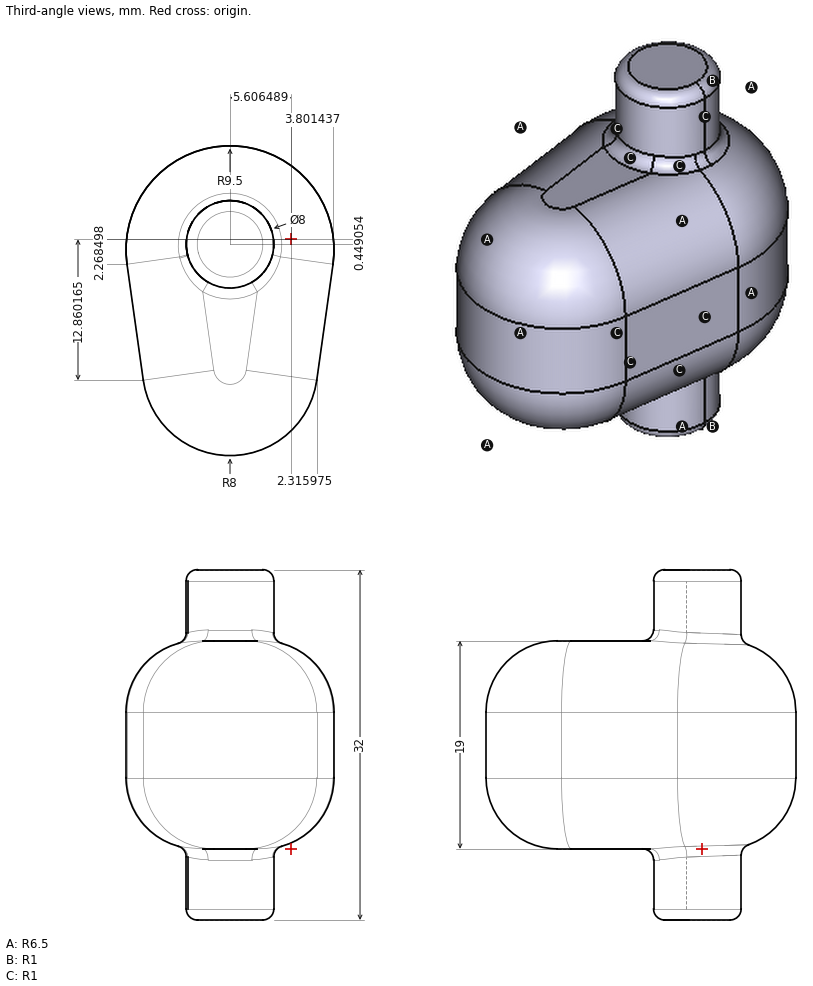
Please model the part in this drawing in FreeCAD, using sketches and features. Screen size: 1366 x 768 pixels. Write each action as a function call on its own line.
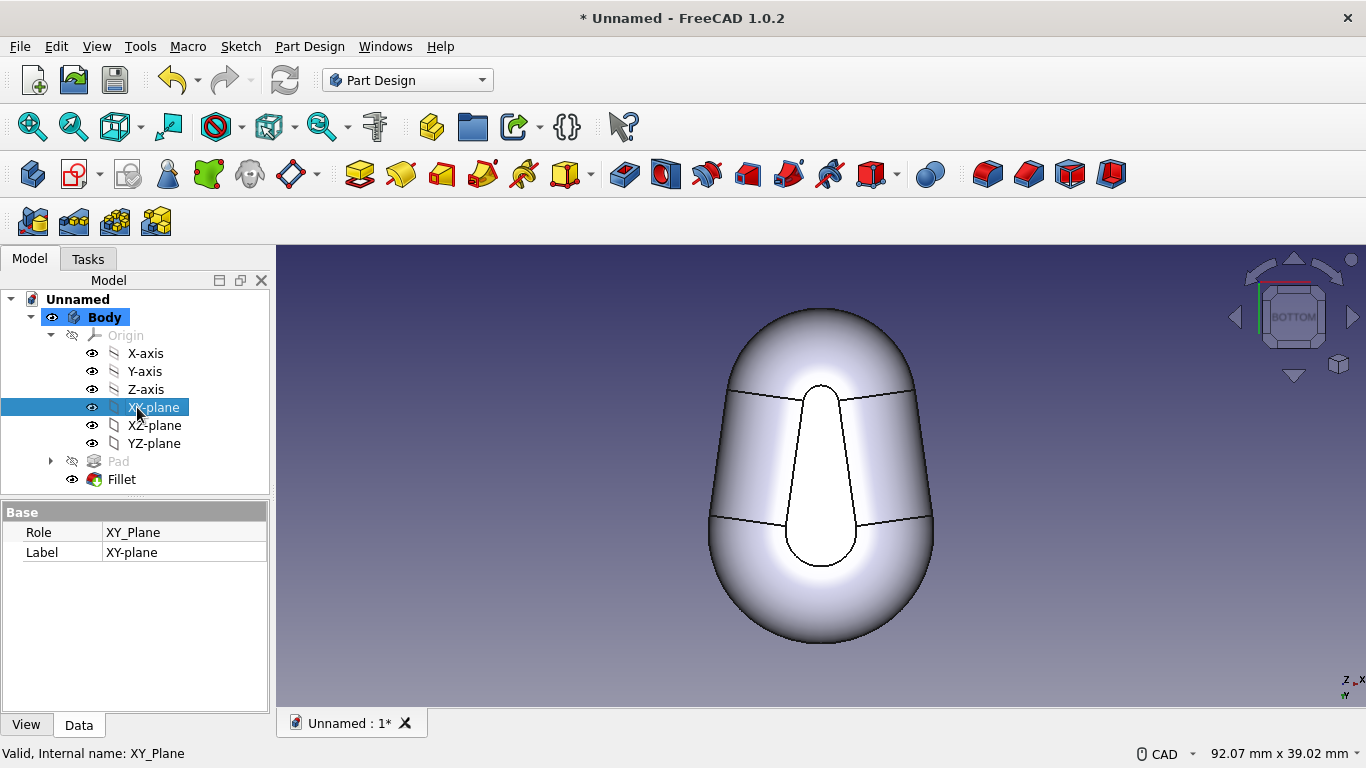
click(290, 174)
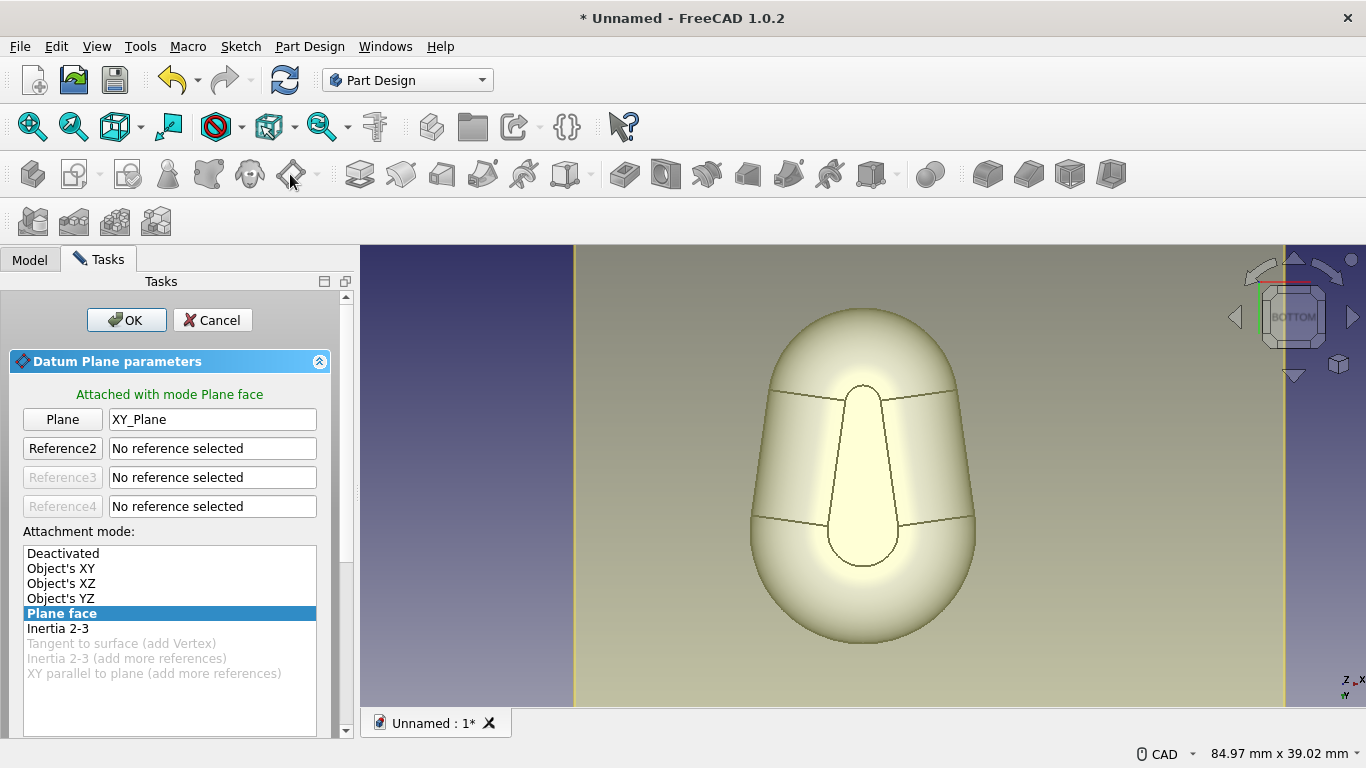
scroll(346, 514, down, 4)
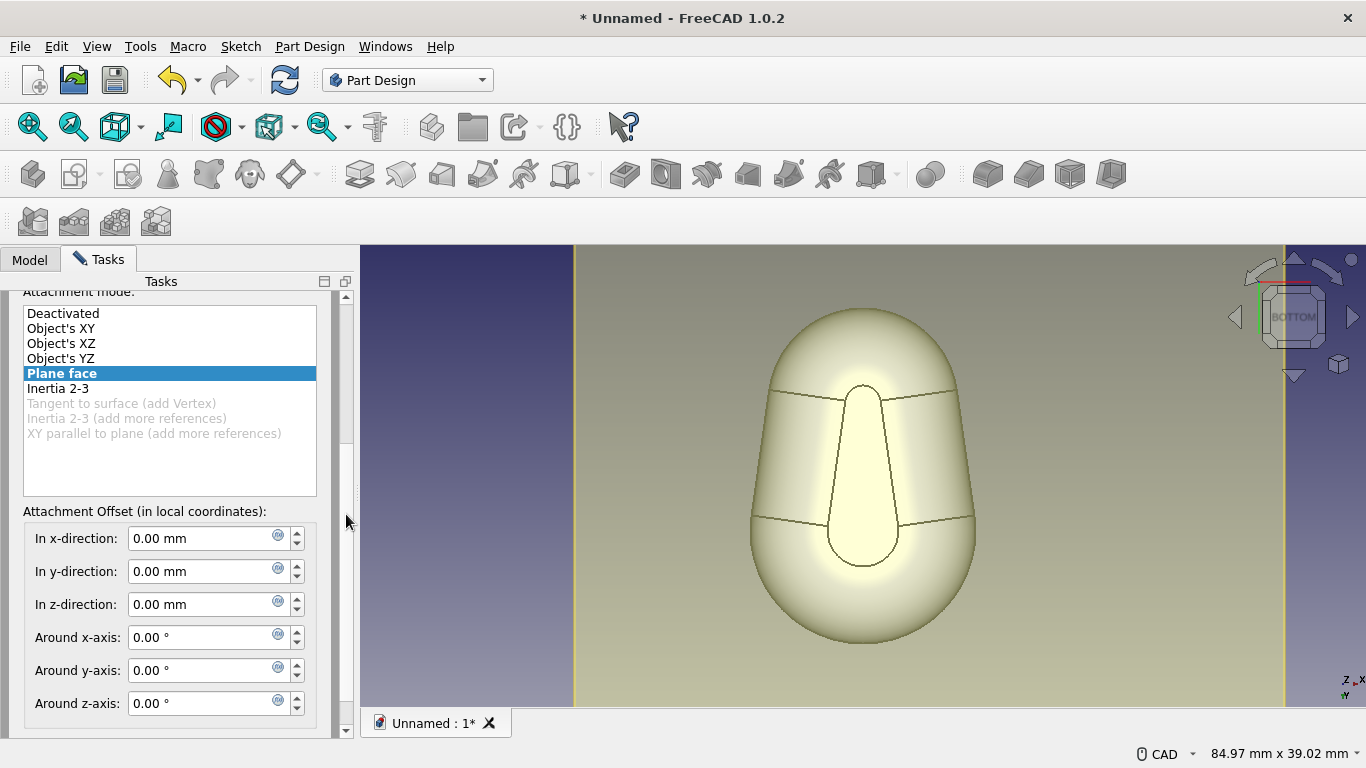
triple_click(210, 604)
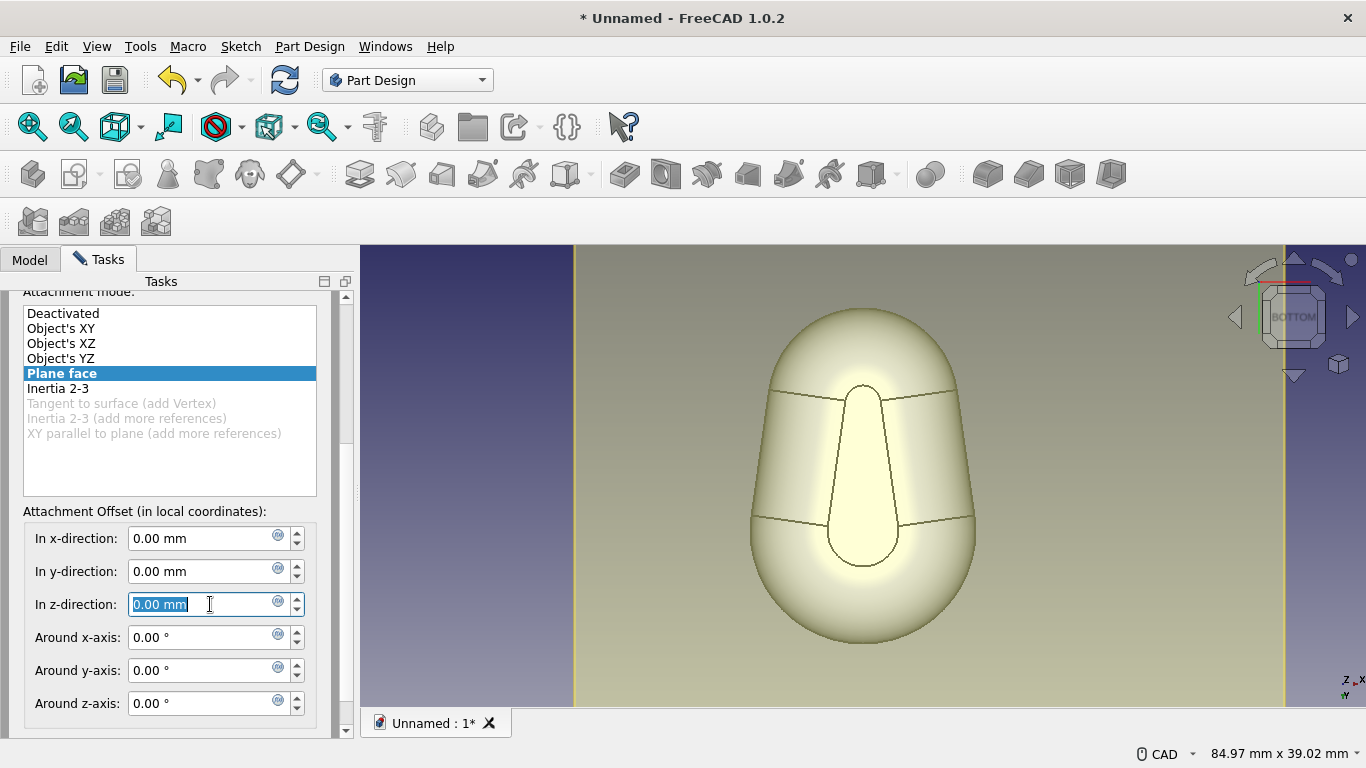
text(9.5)
key(Tab)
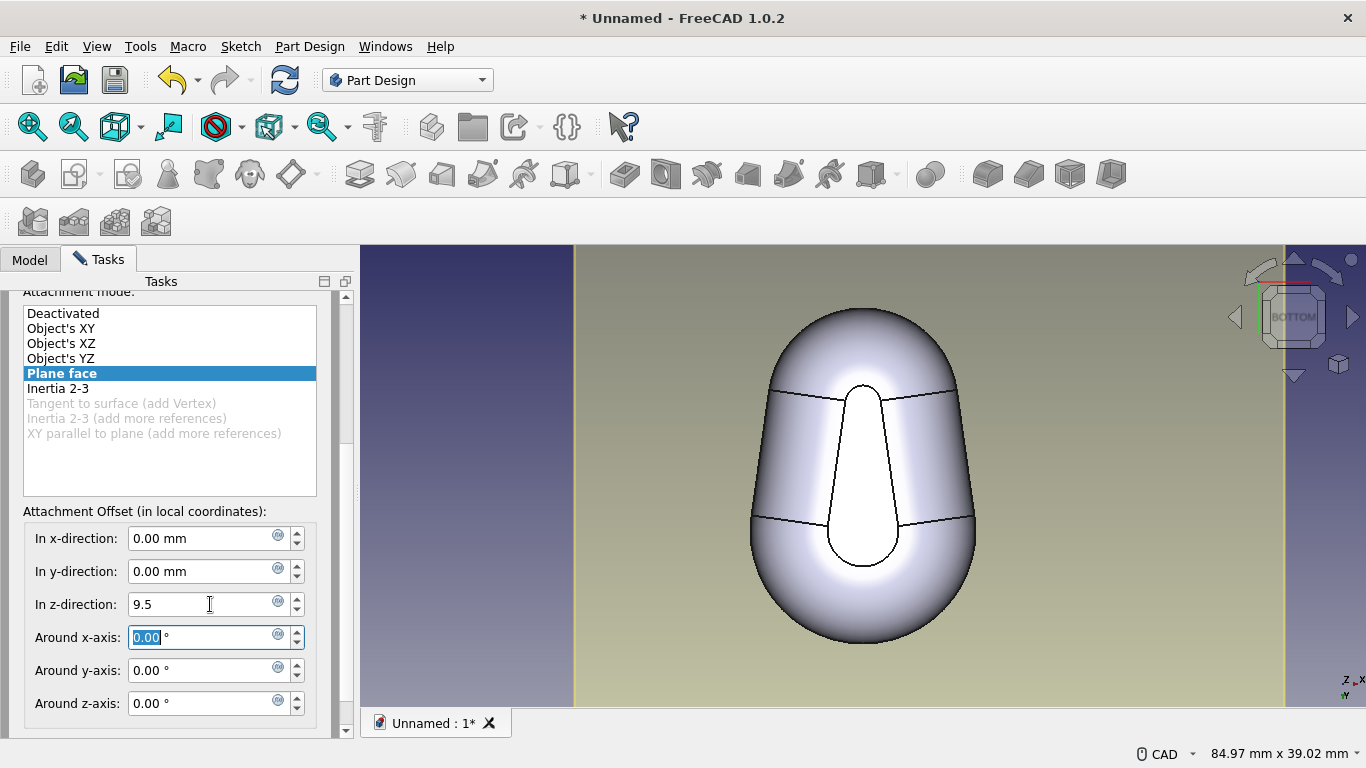
scroll(346, 514, up, 5)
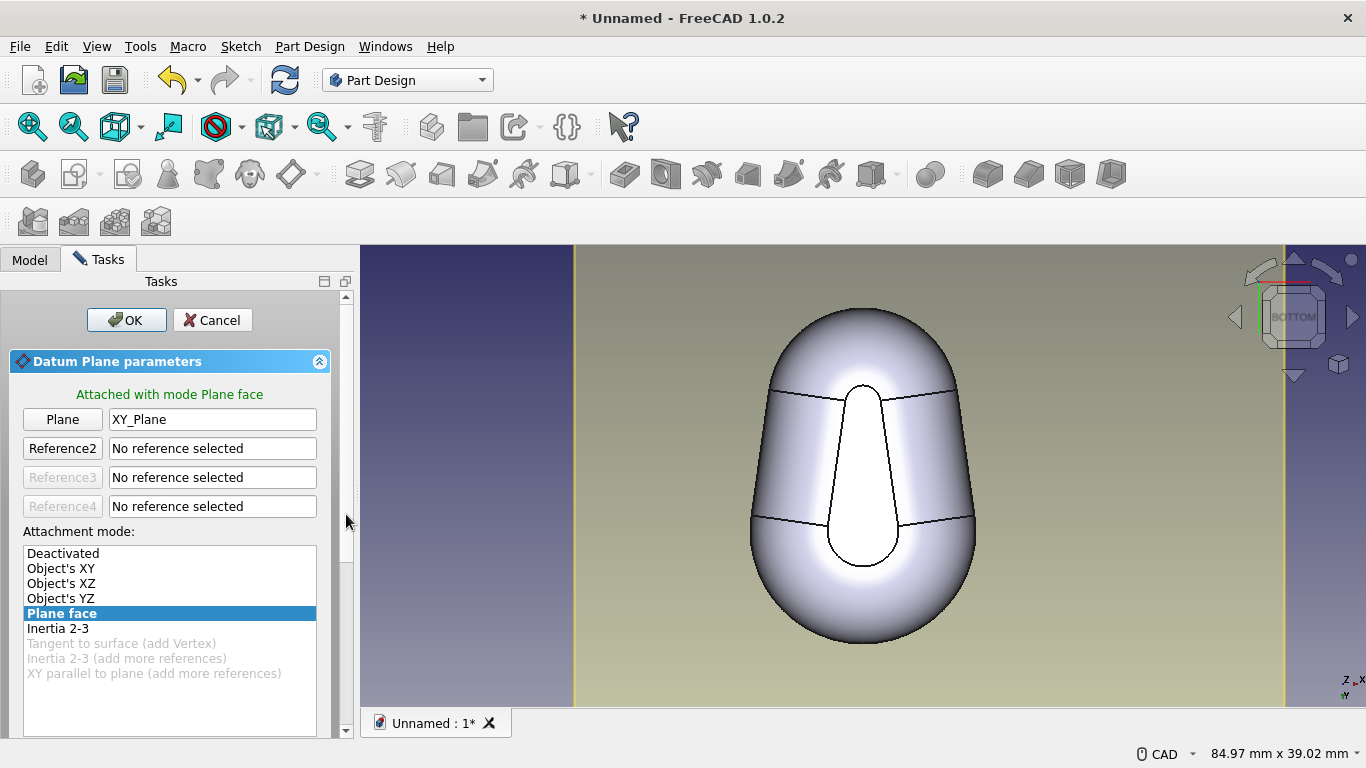
click(127, 320)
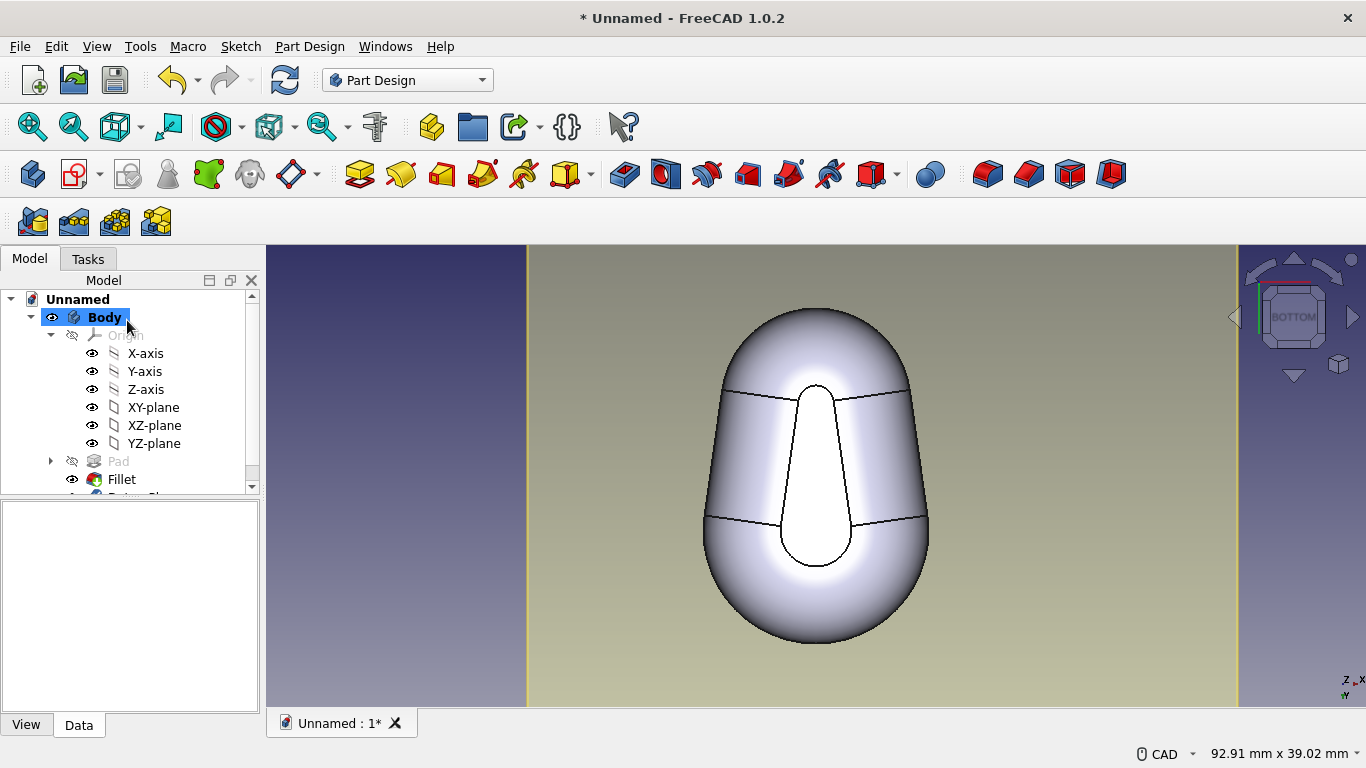
scroll(101, 385, down, 3)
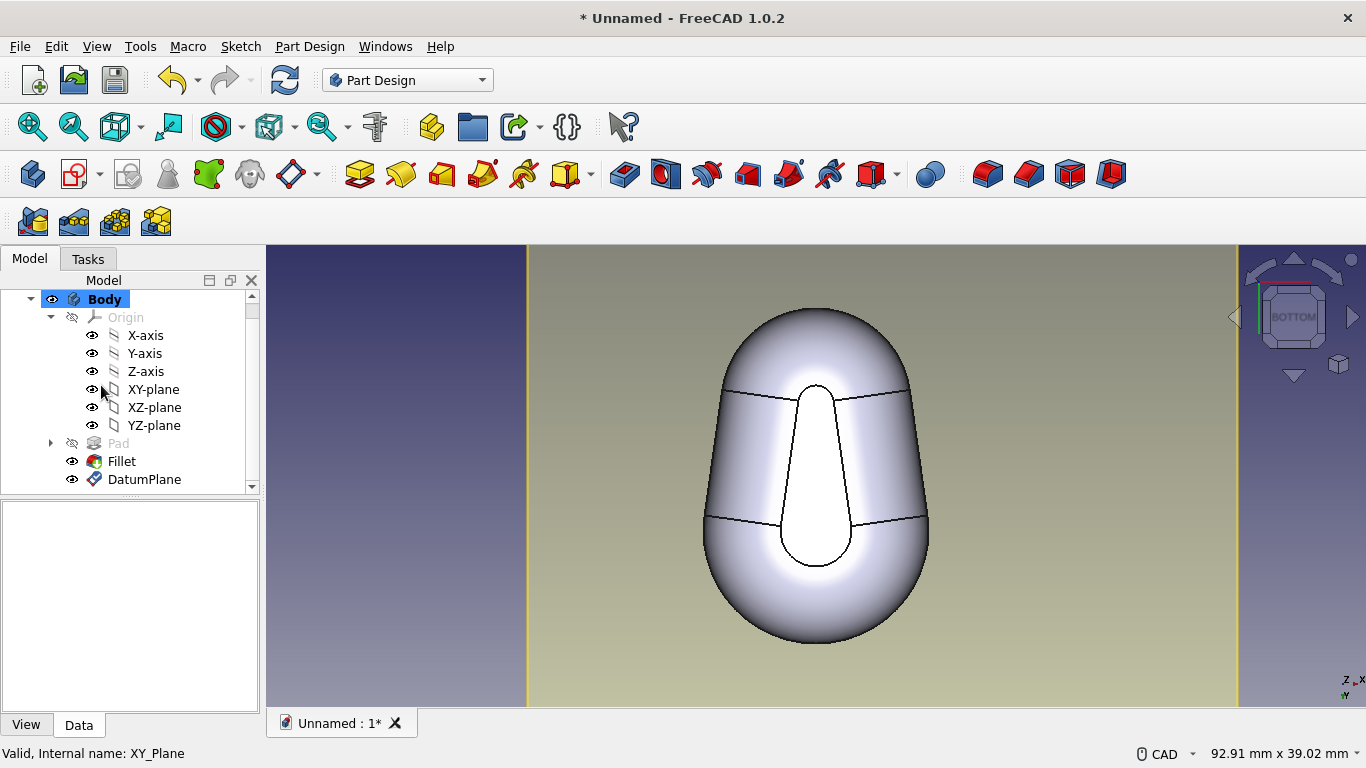
click(117, 479)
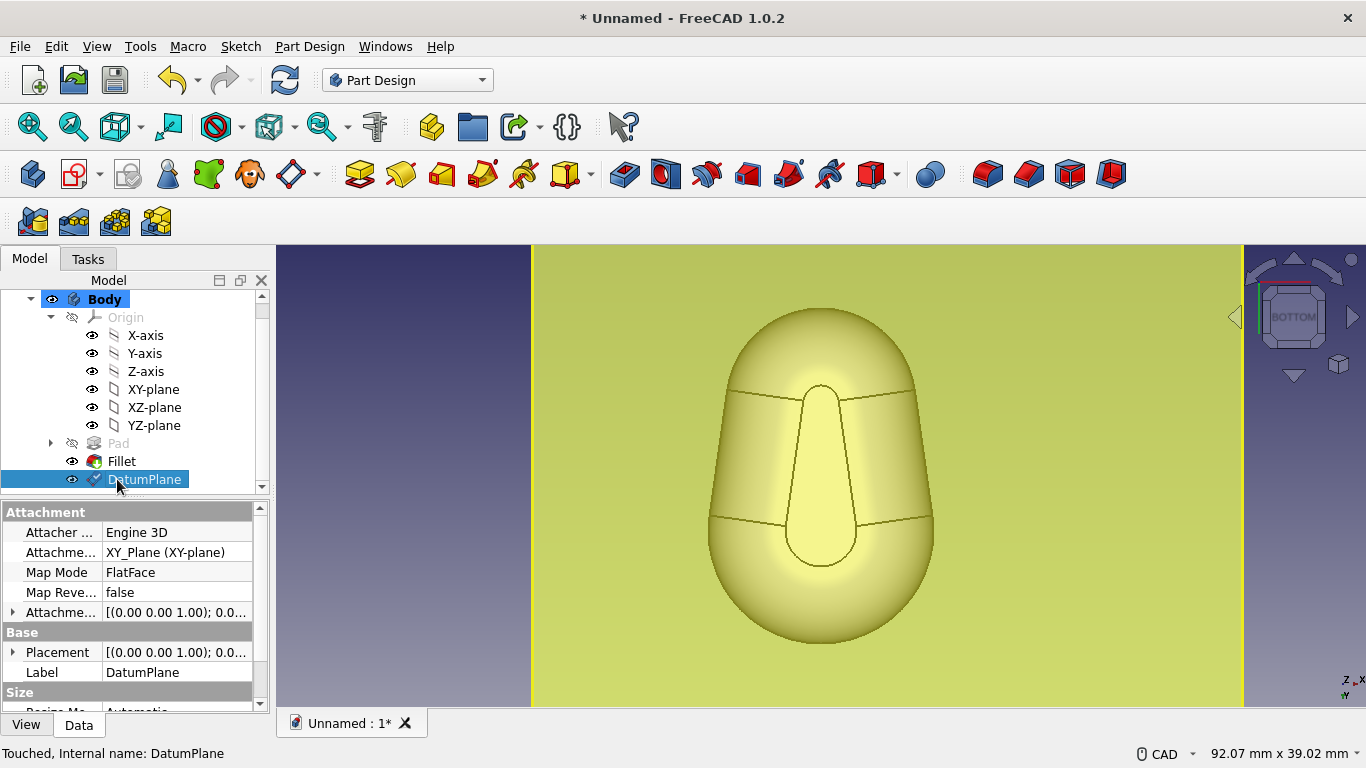
click(74, 174)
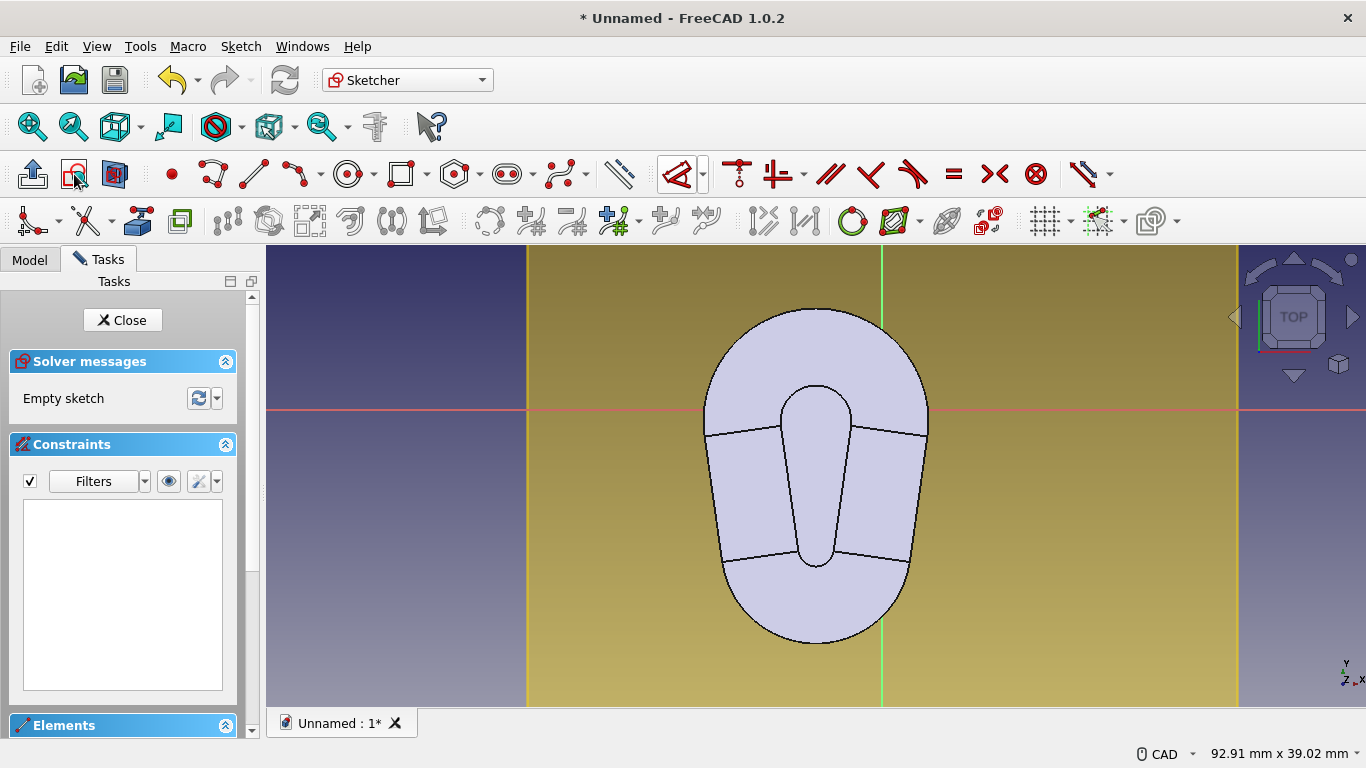
click(115, 174)